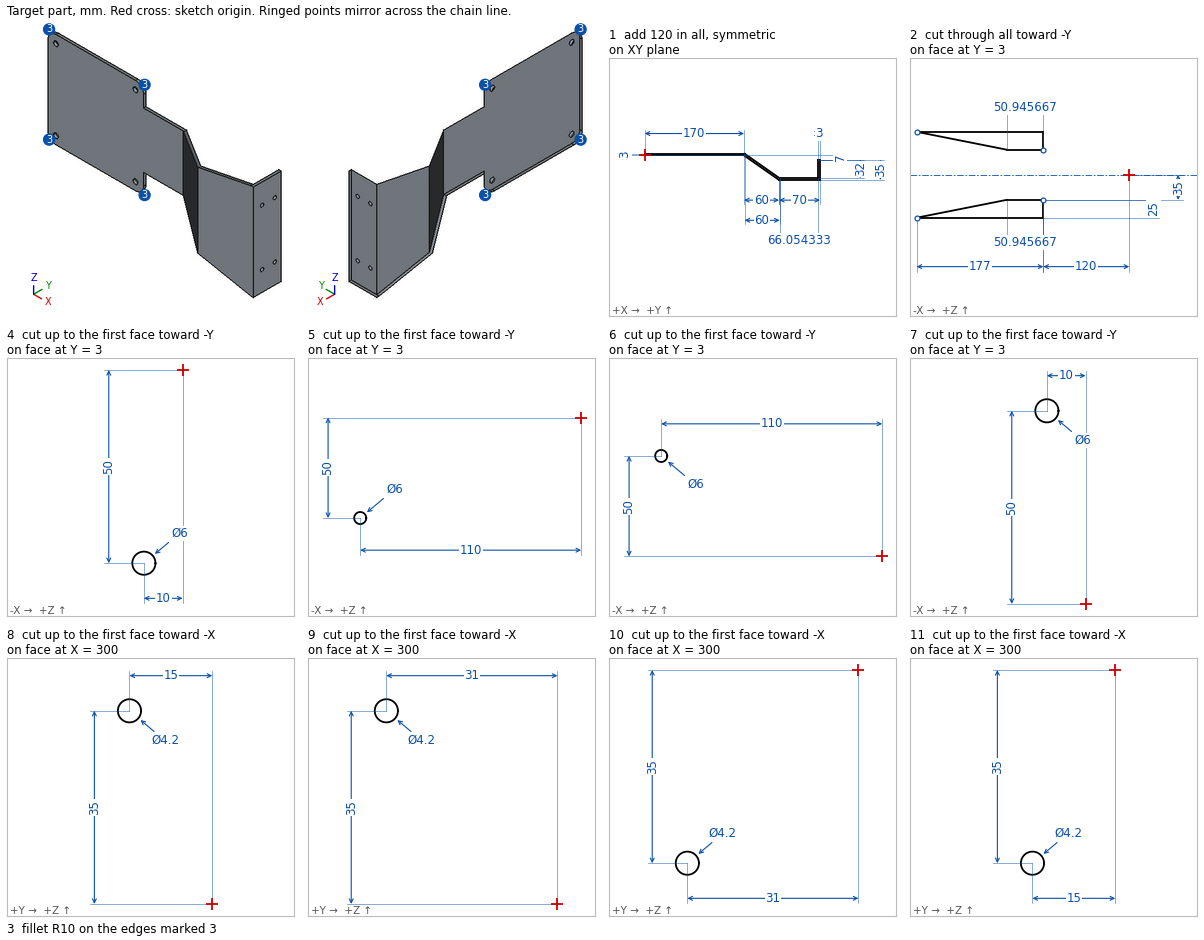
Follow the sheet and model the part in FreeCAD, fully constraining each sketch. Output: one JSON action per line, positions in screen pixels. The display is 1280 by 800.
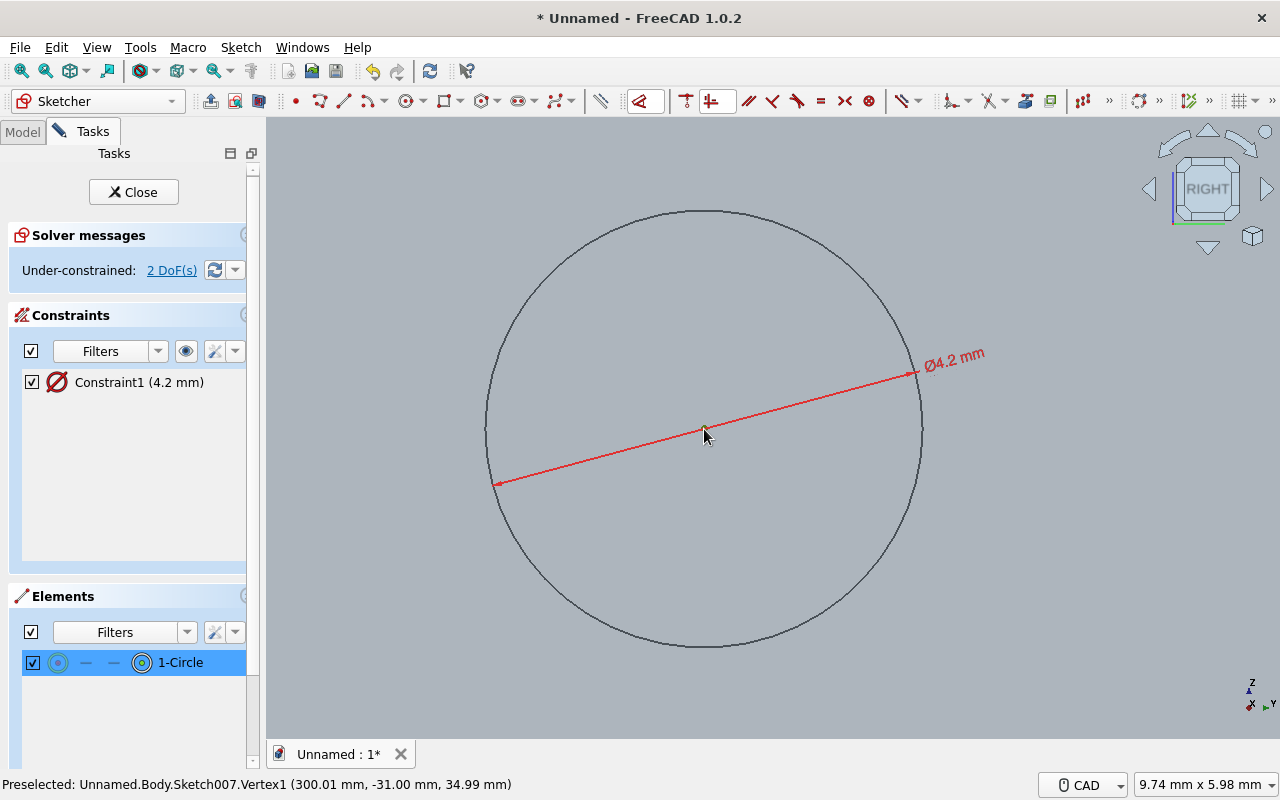
{"action": "key", "text": "l"}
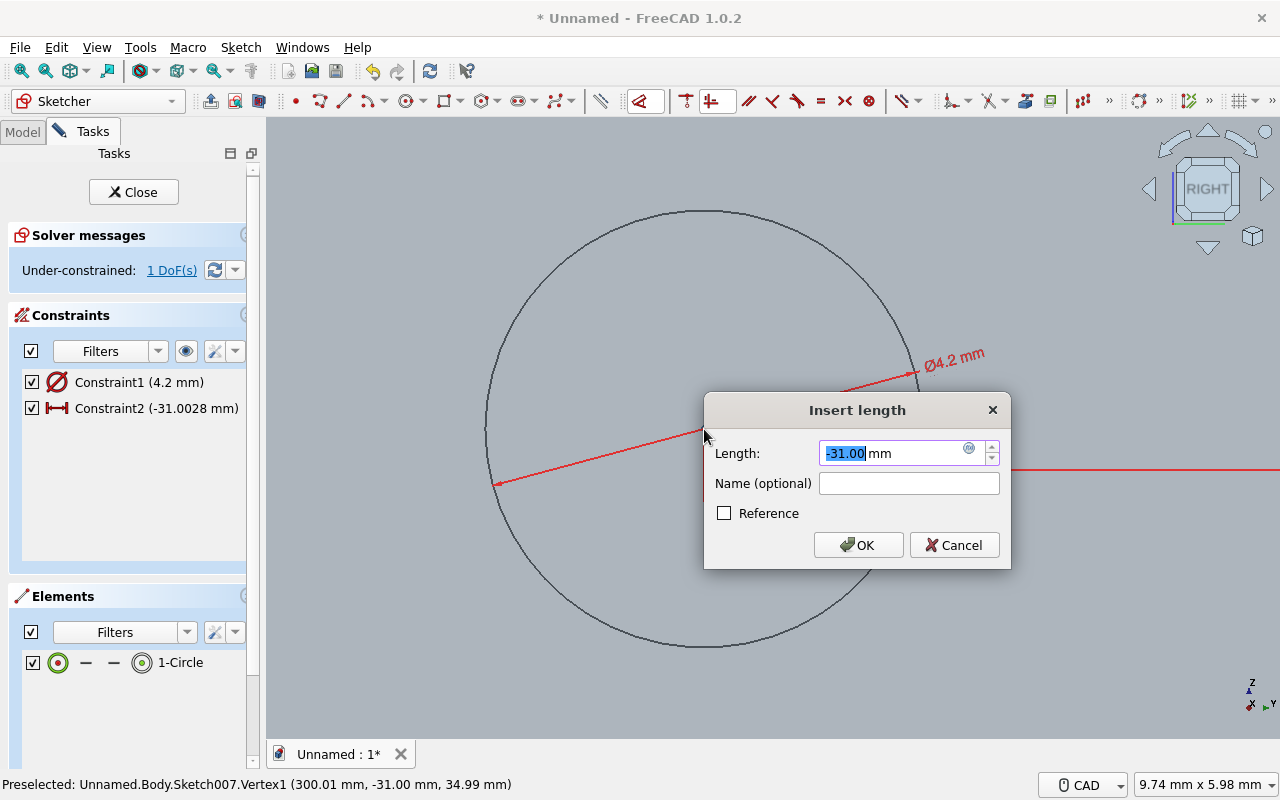
{"action": "type", "text": "-31"}
{"action": "key", "text": "Return"}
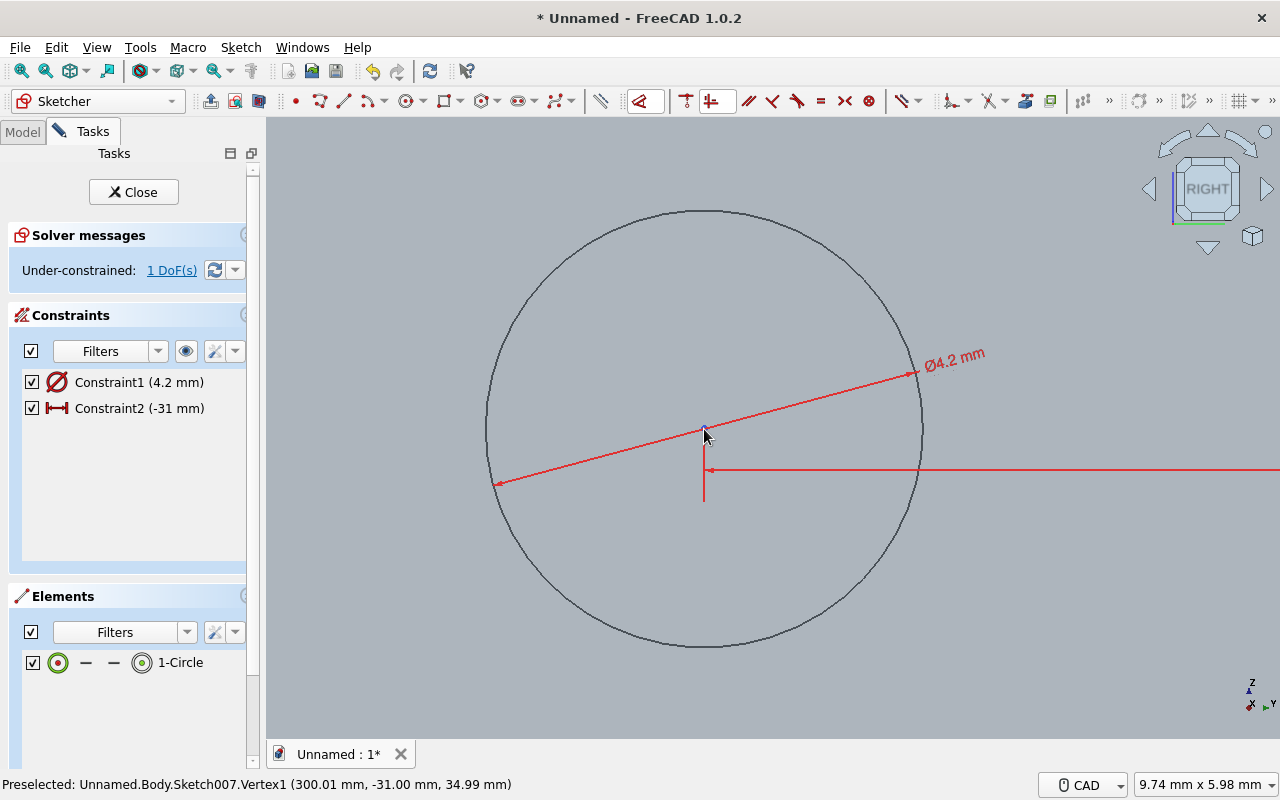
{"action": "left_click", "coordinate": [704, 429]}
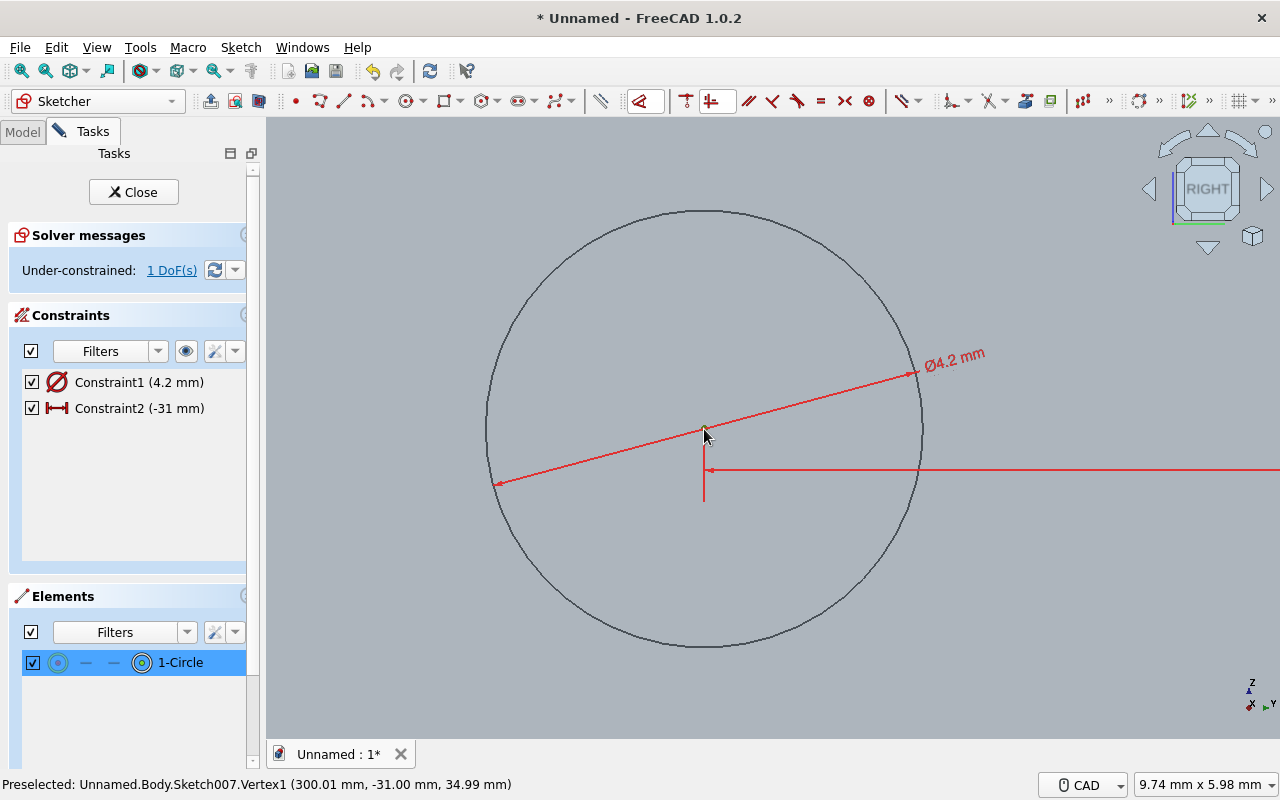
{"action": "left_click", "coordinate": [658, 102]}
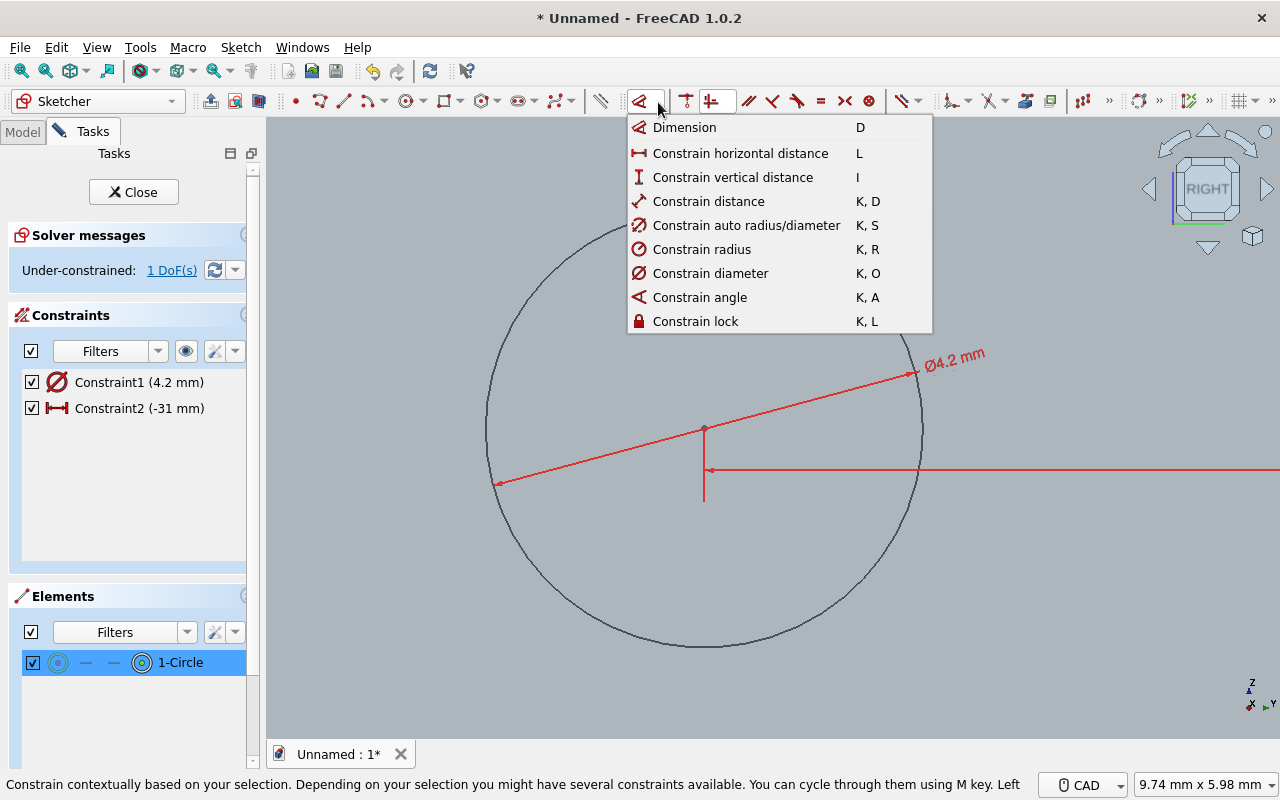
{"action": "left_click", "coordinate": [780, 177]}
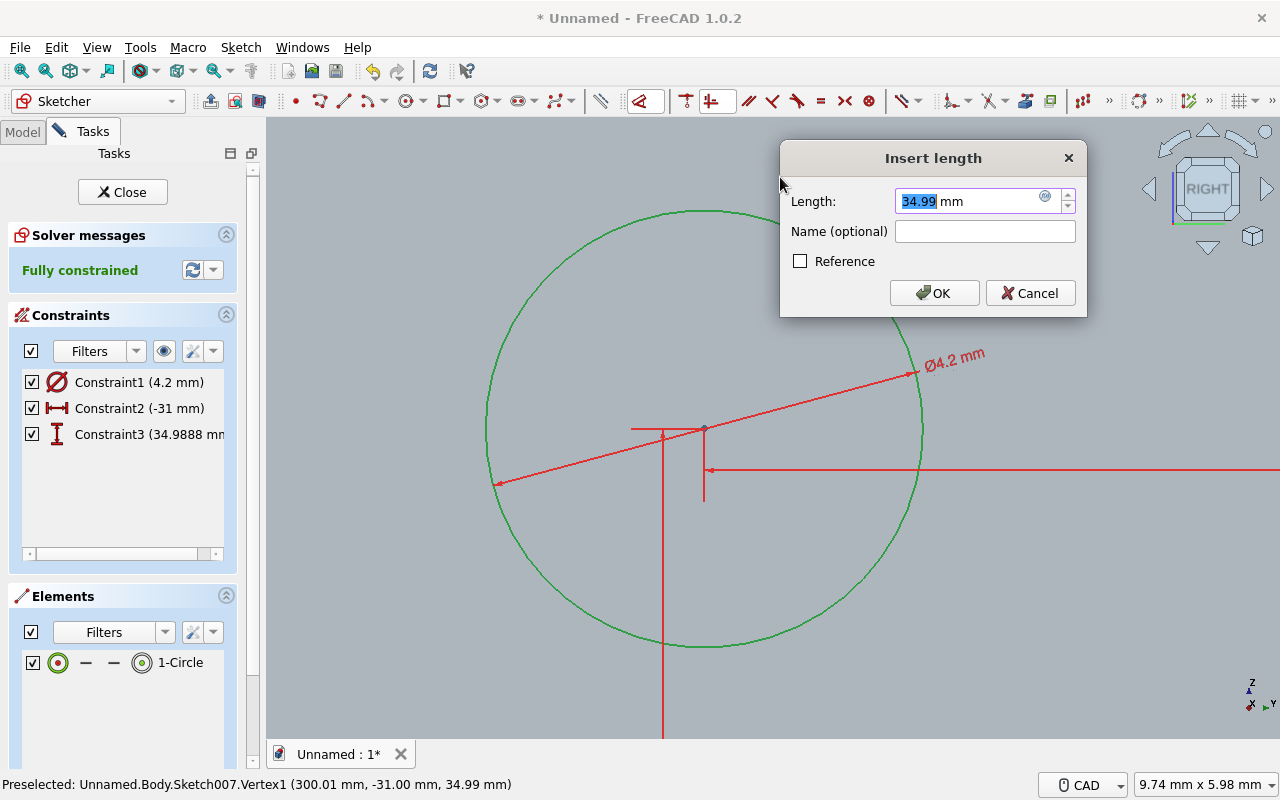
{"action": "type", "text": "35"}
{"action": "key", "text": "Return"}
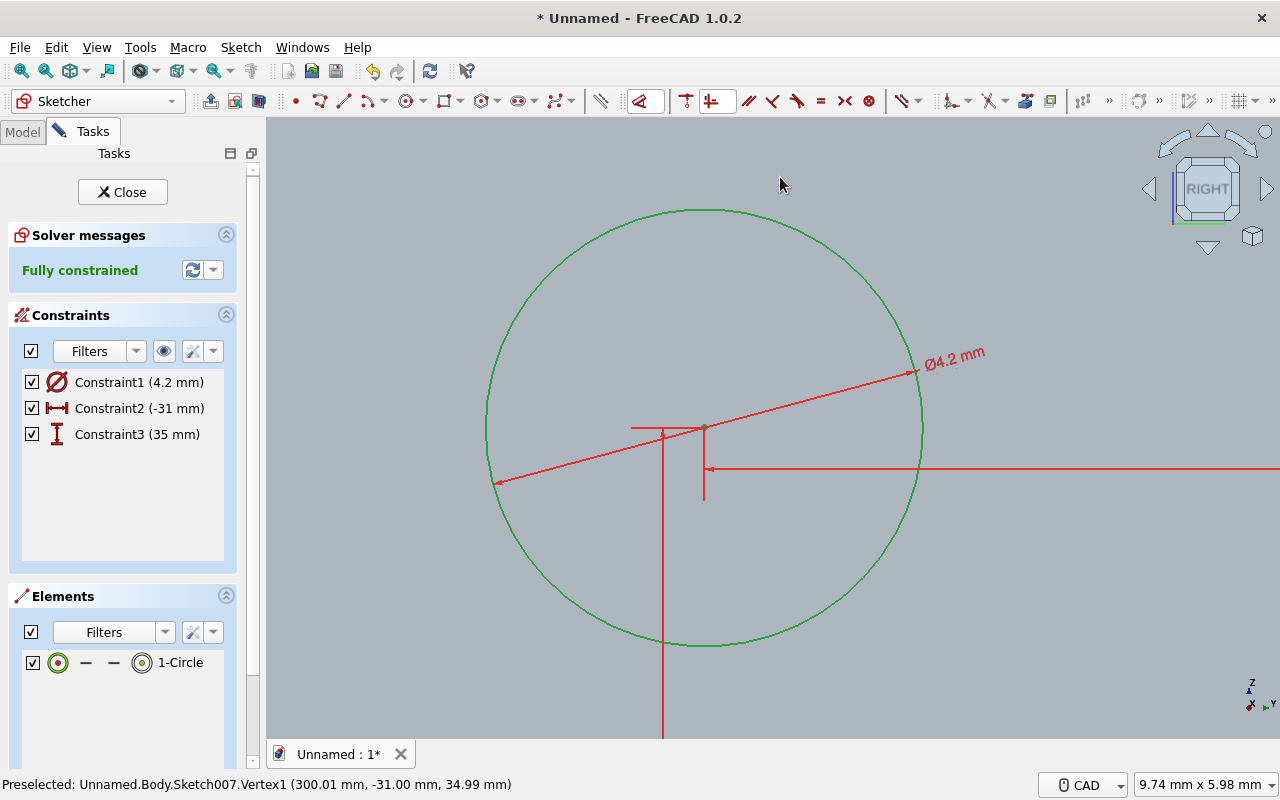
{"action": "left_click", "coordinate": [123, 192]}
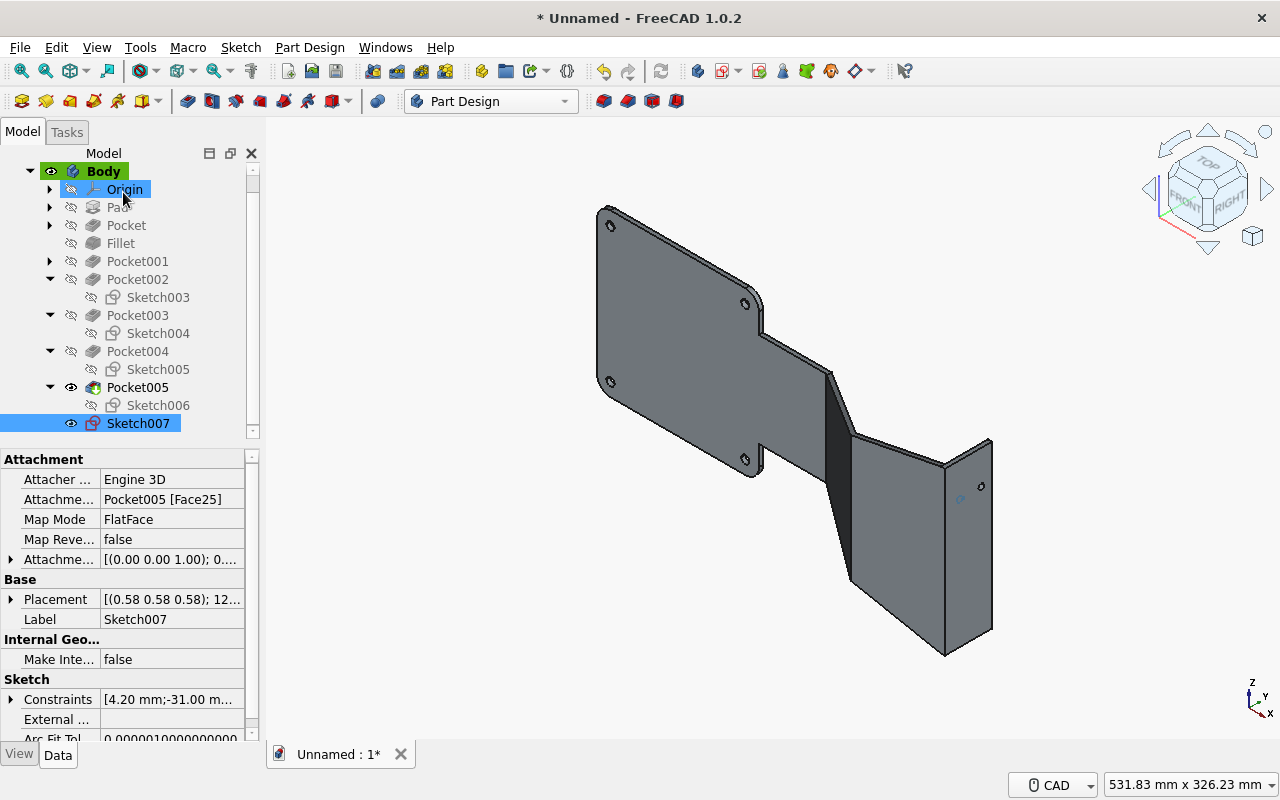
{"action": "left_click", "coordinate": [188, 102]}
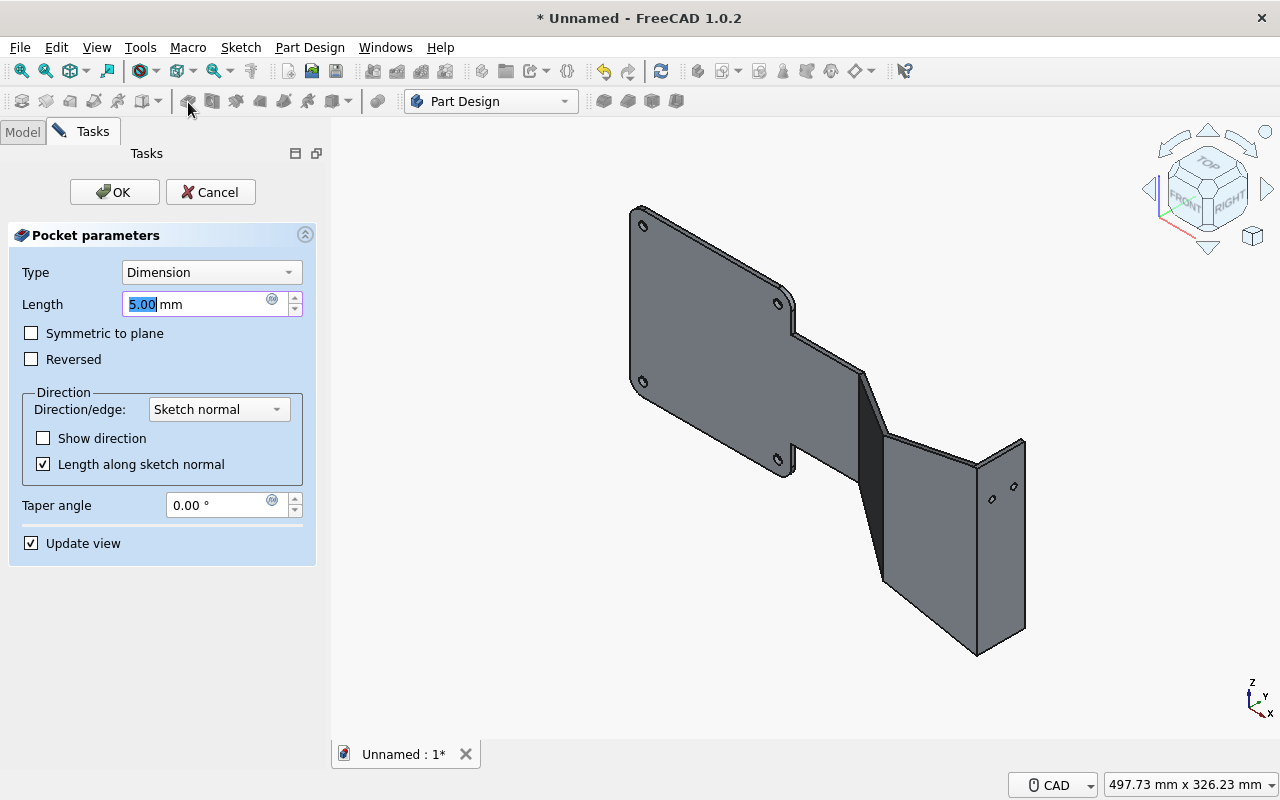
{"action": "left_click", "coordinate": [212, 272]}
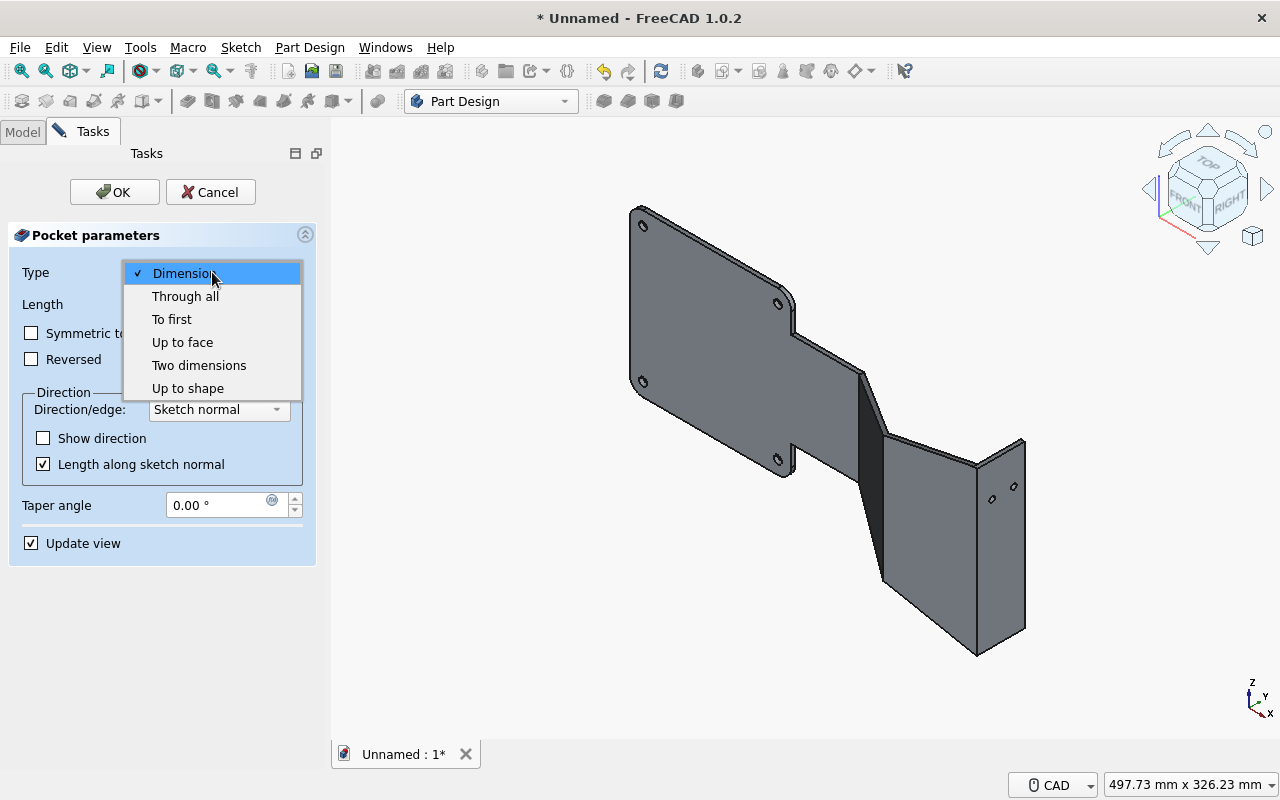
{"action": "left_click", "coordinate": [212, 320]}